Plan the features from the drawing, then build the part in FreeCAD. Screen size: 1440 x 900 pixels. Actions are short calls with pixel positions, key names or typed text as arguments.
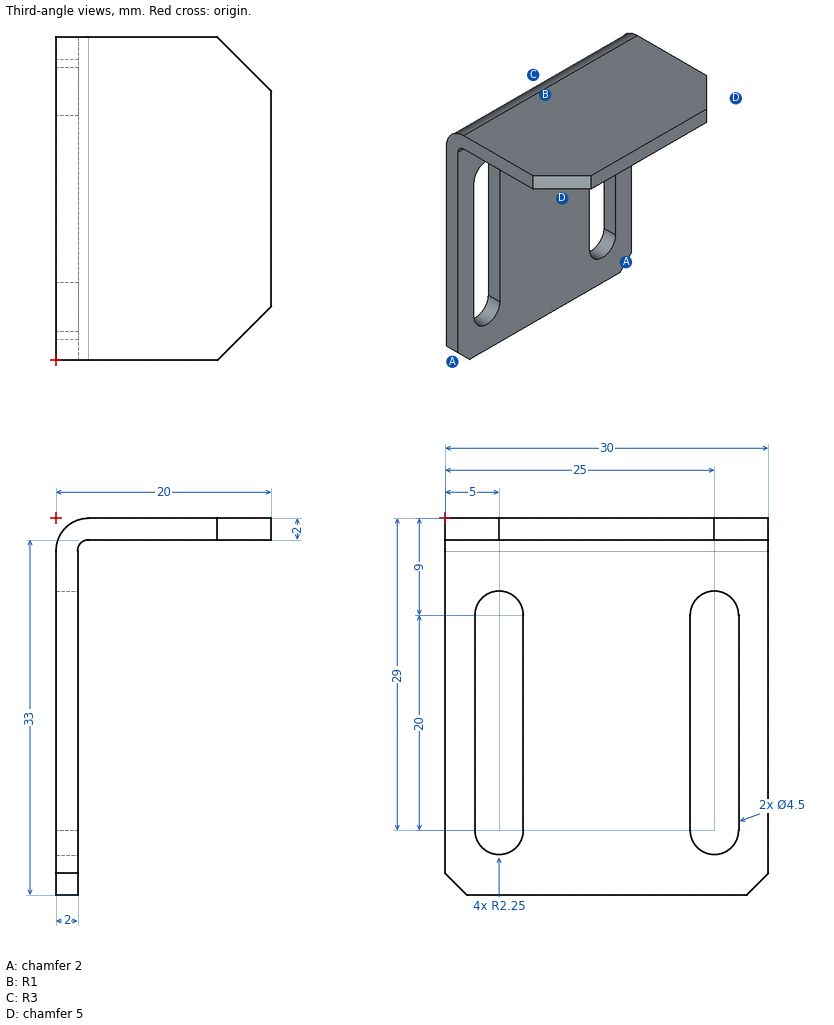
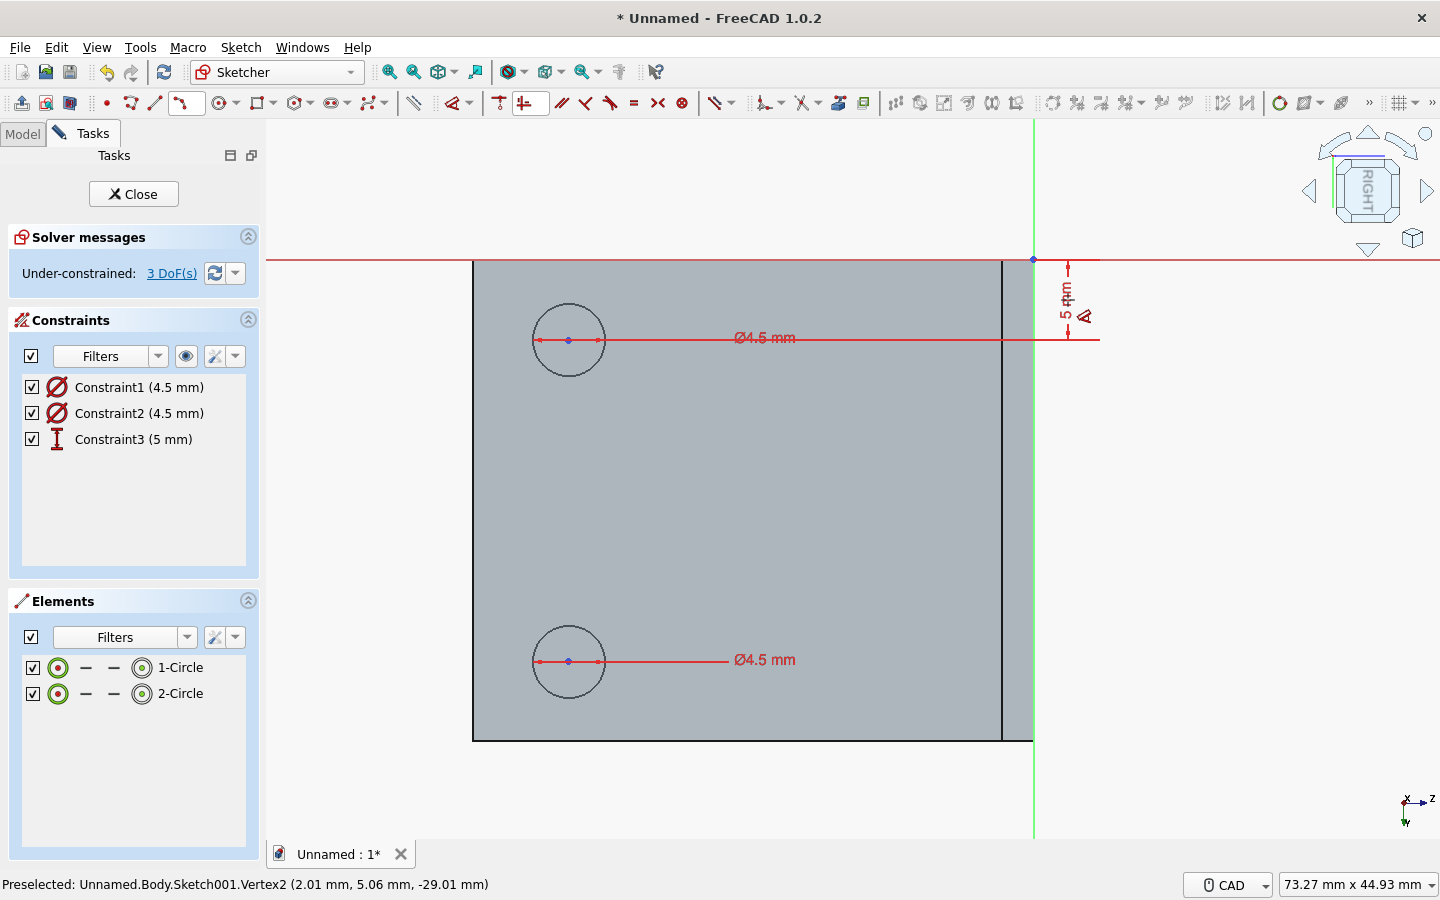
click(569, 662)
click(801, 226)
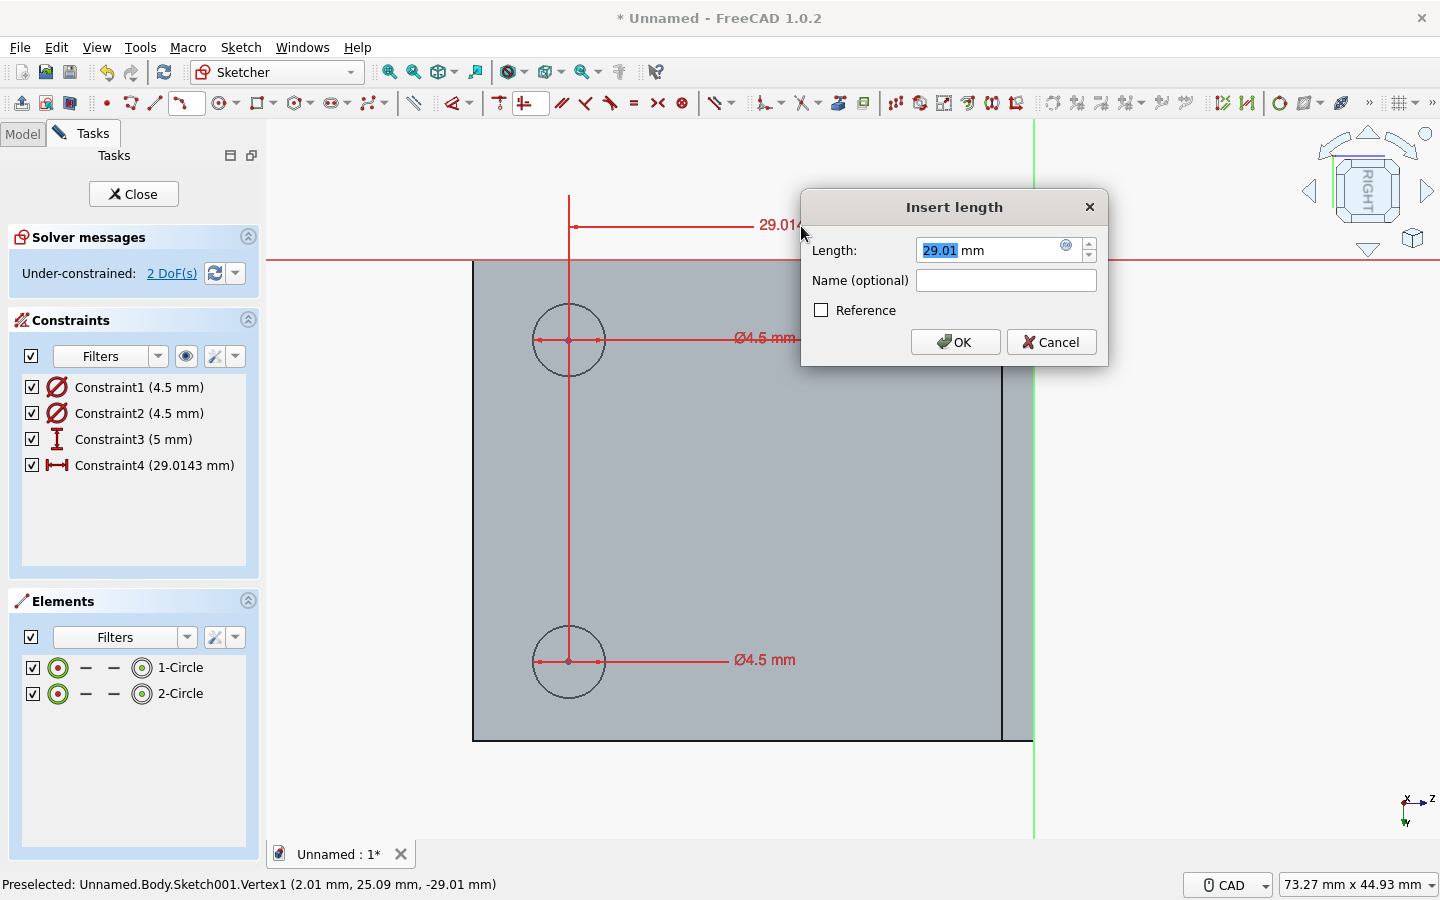
text(29)
key(Return)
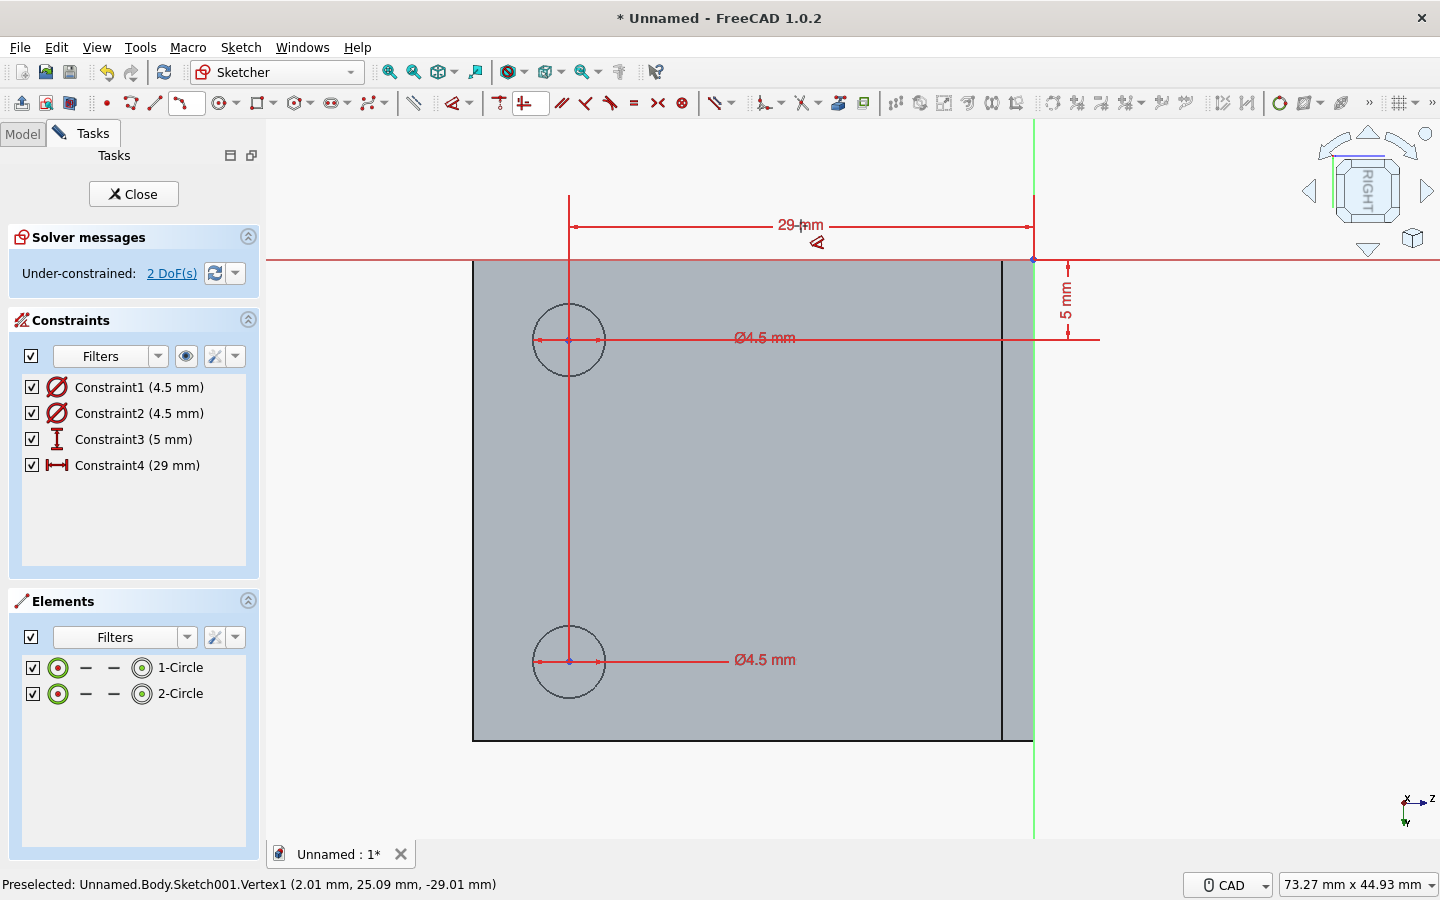
click(569, 662)
click(1068, 461)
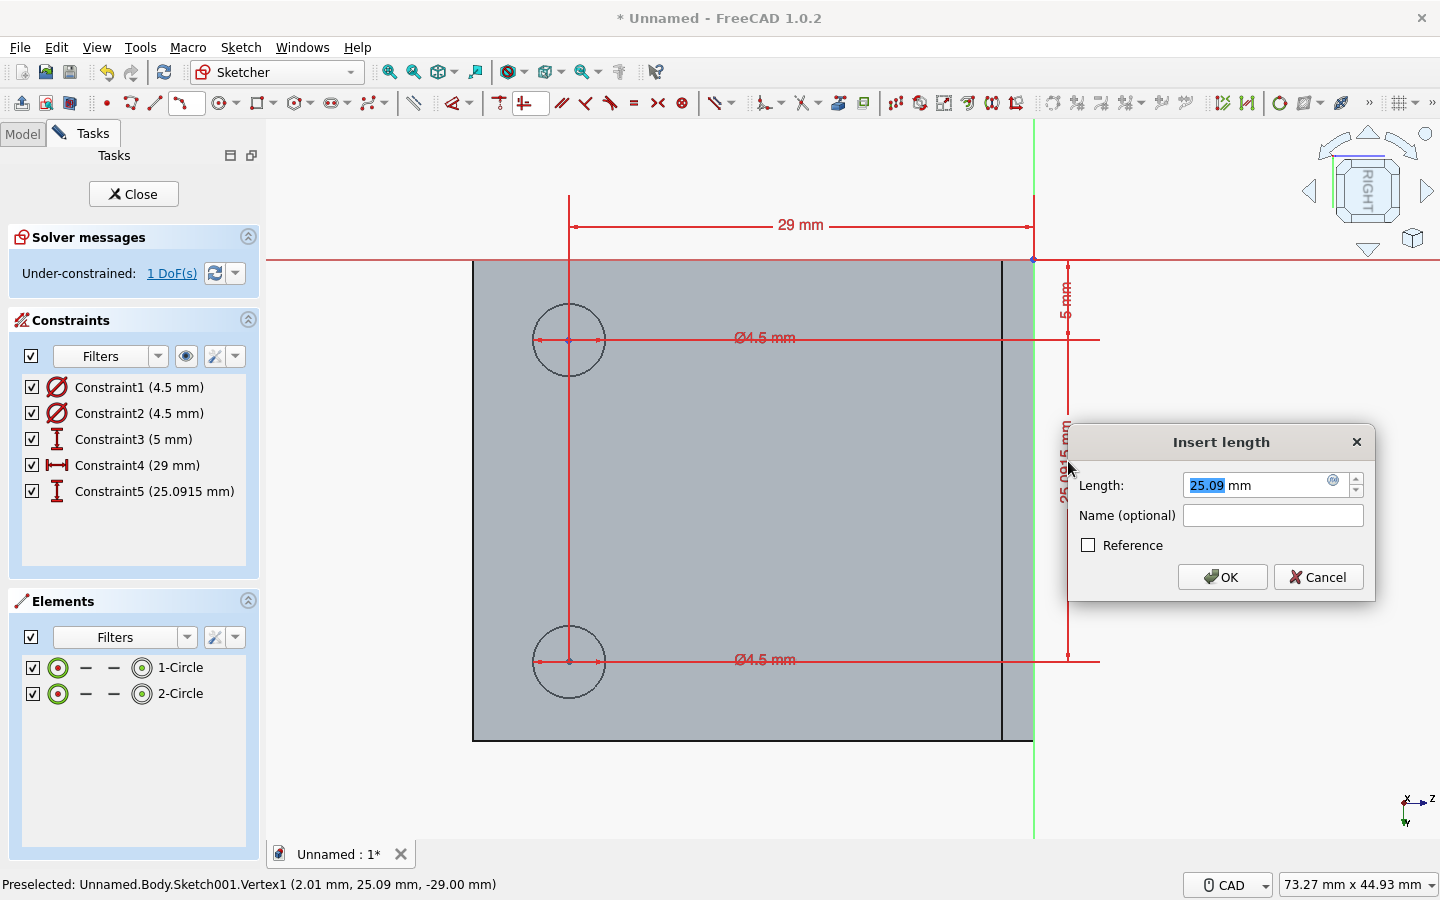
text(25)
key(Return)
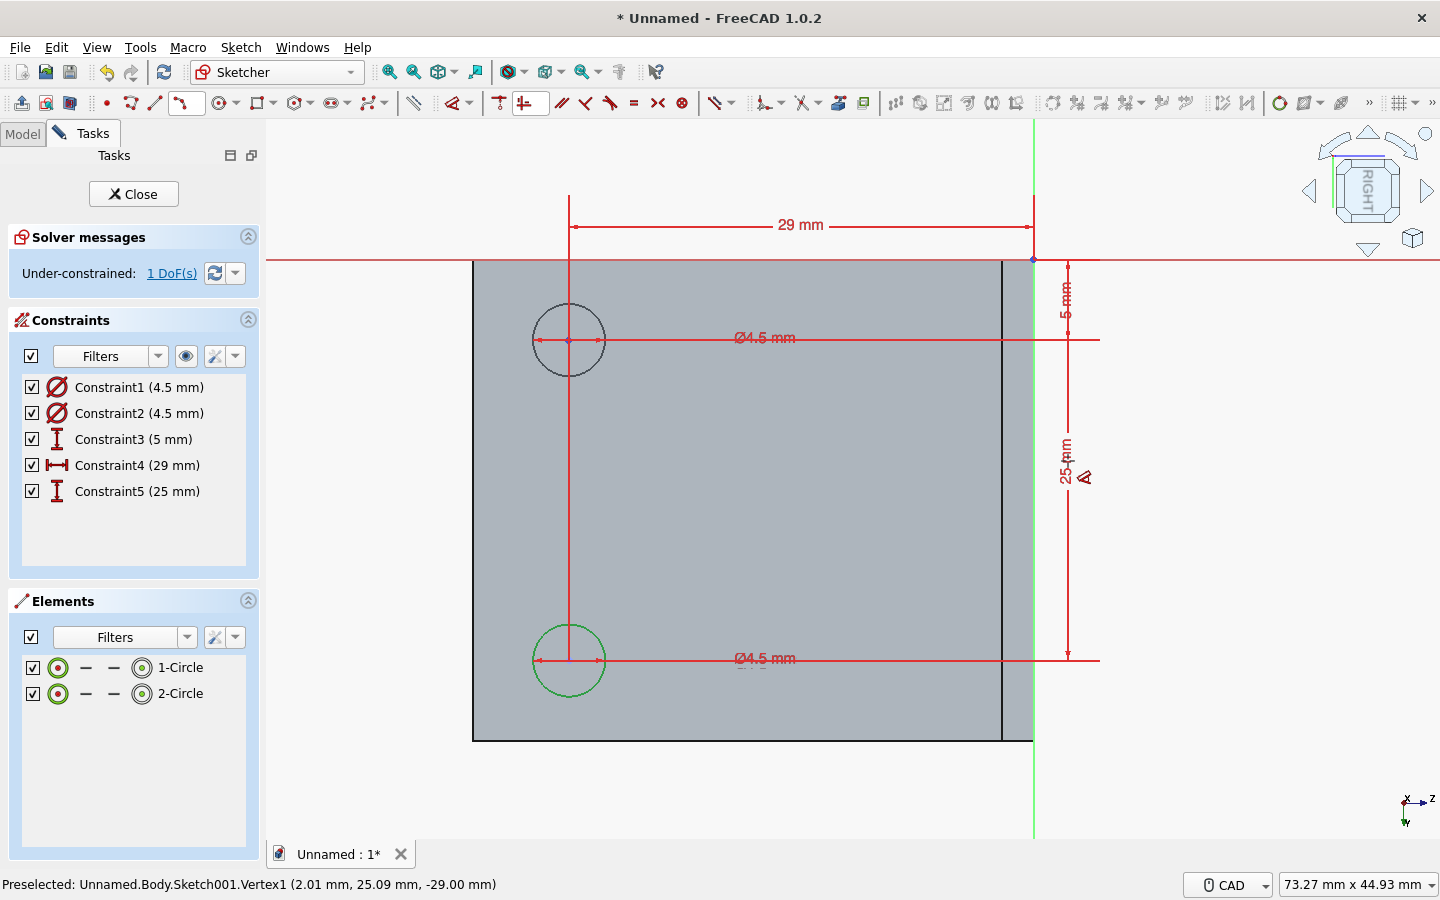
click(569, 340)
click(695, 226)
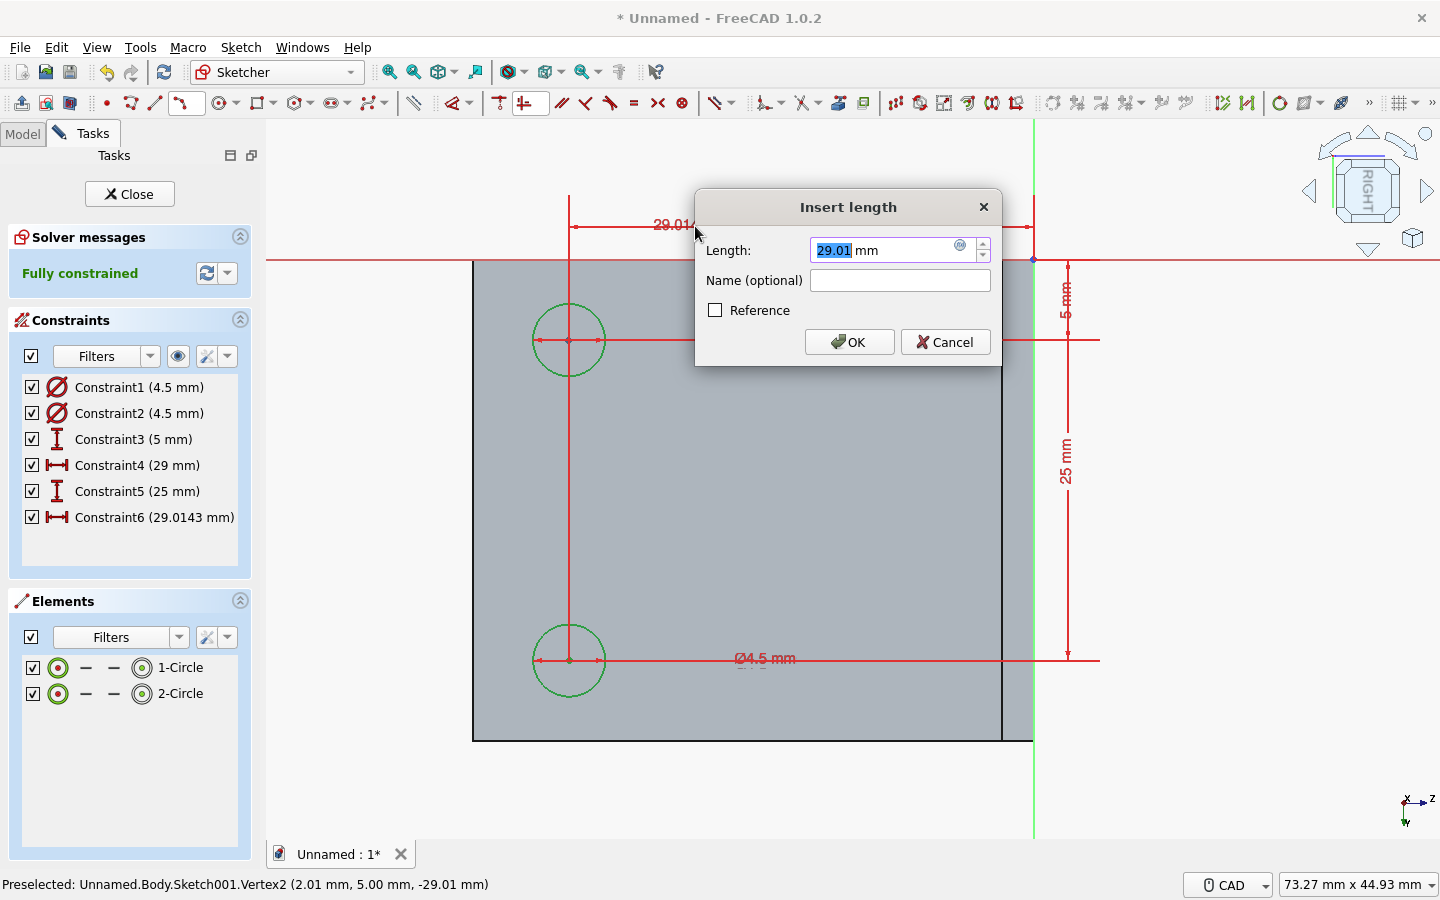
text(29)
key(Return)
key(Escape)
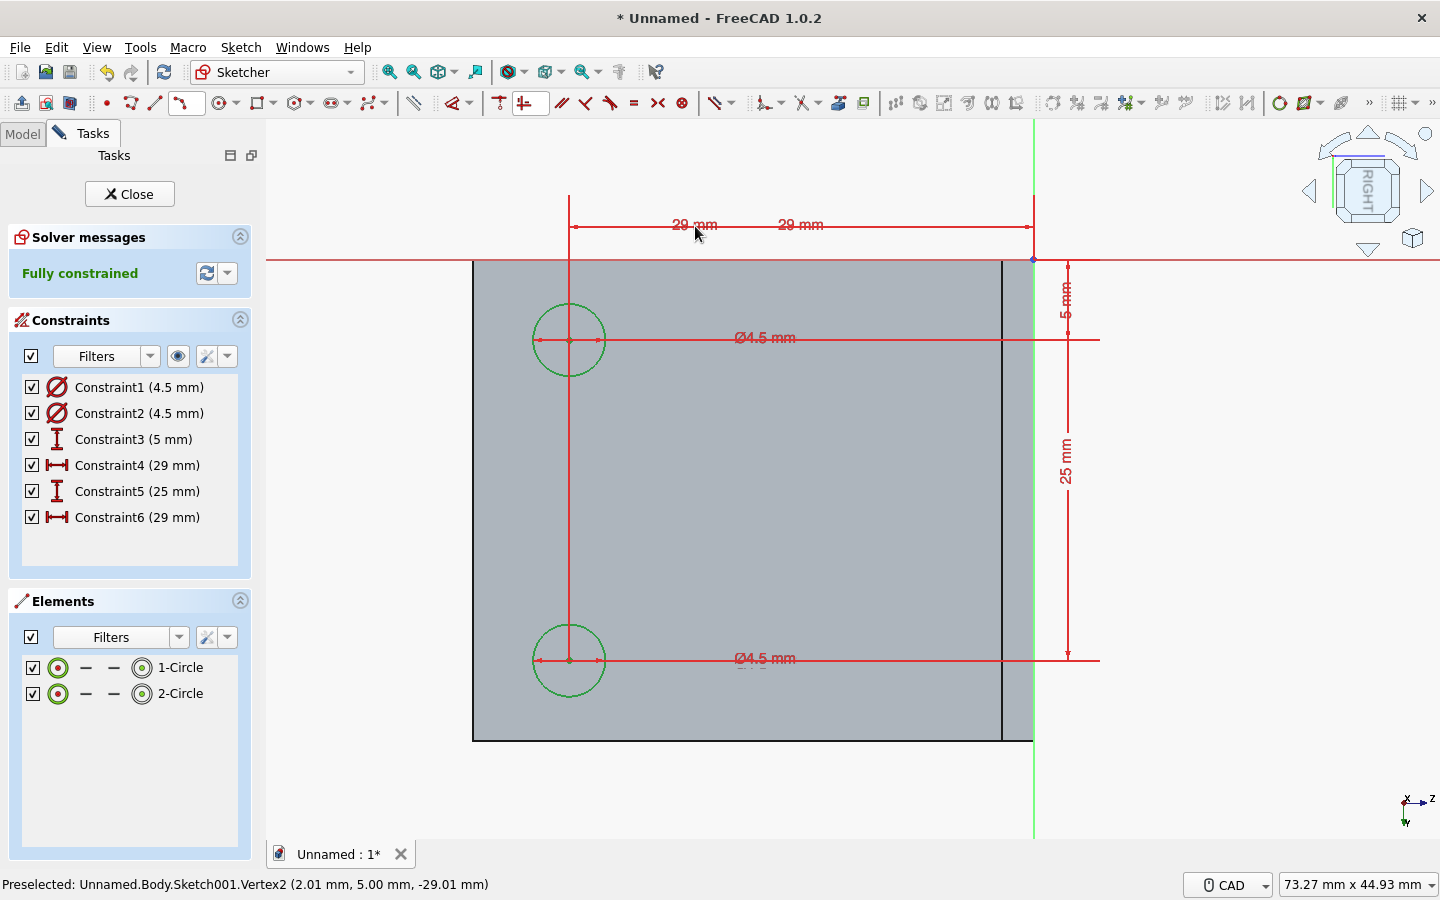
click(130, 194)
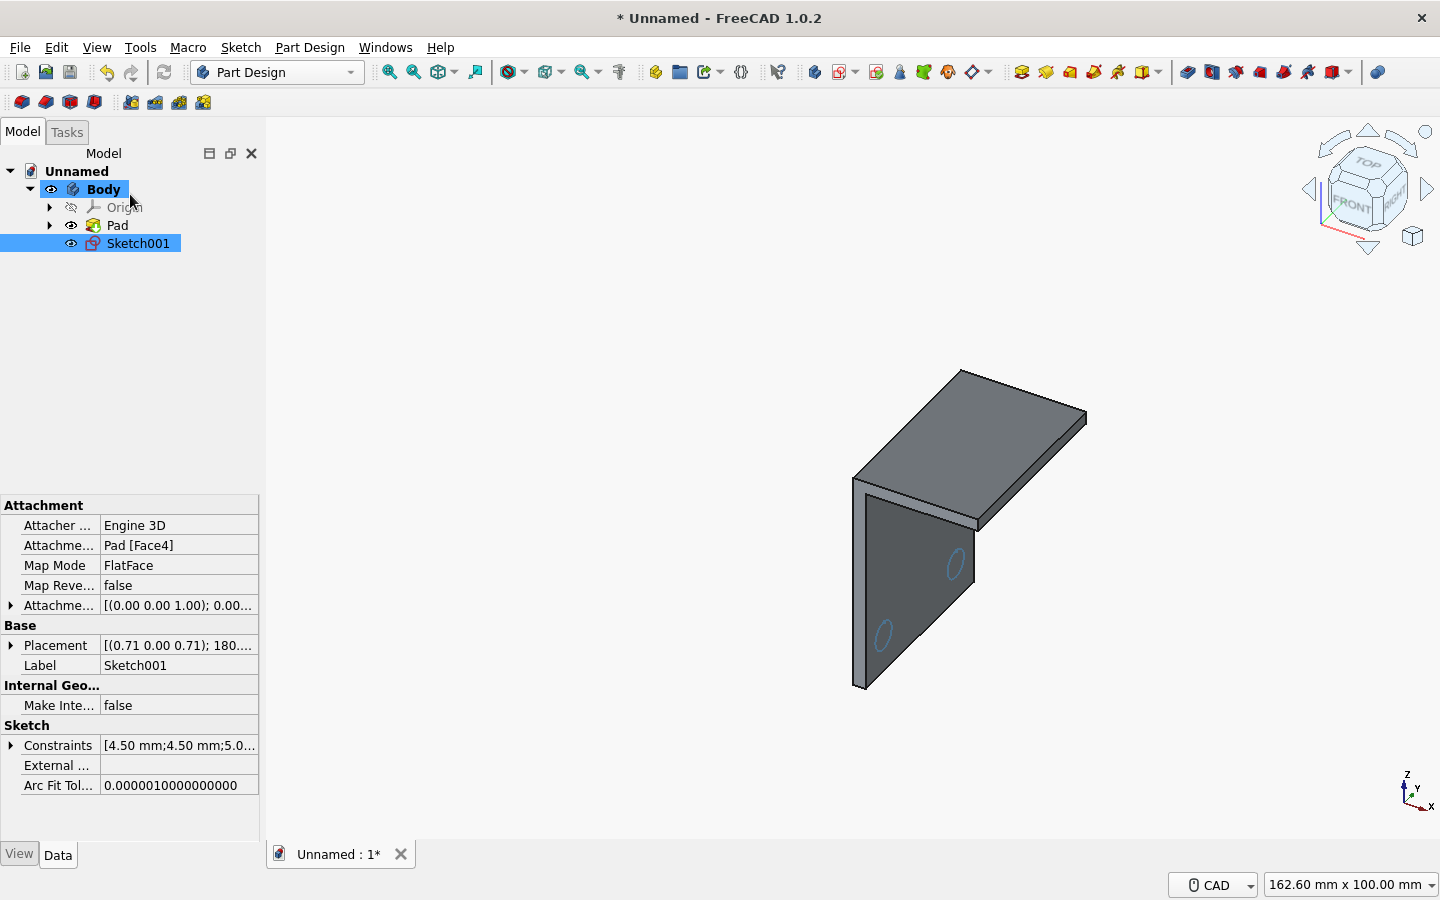
click(1188, 72)